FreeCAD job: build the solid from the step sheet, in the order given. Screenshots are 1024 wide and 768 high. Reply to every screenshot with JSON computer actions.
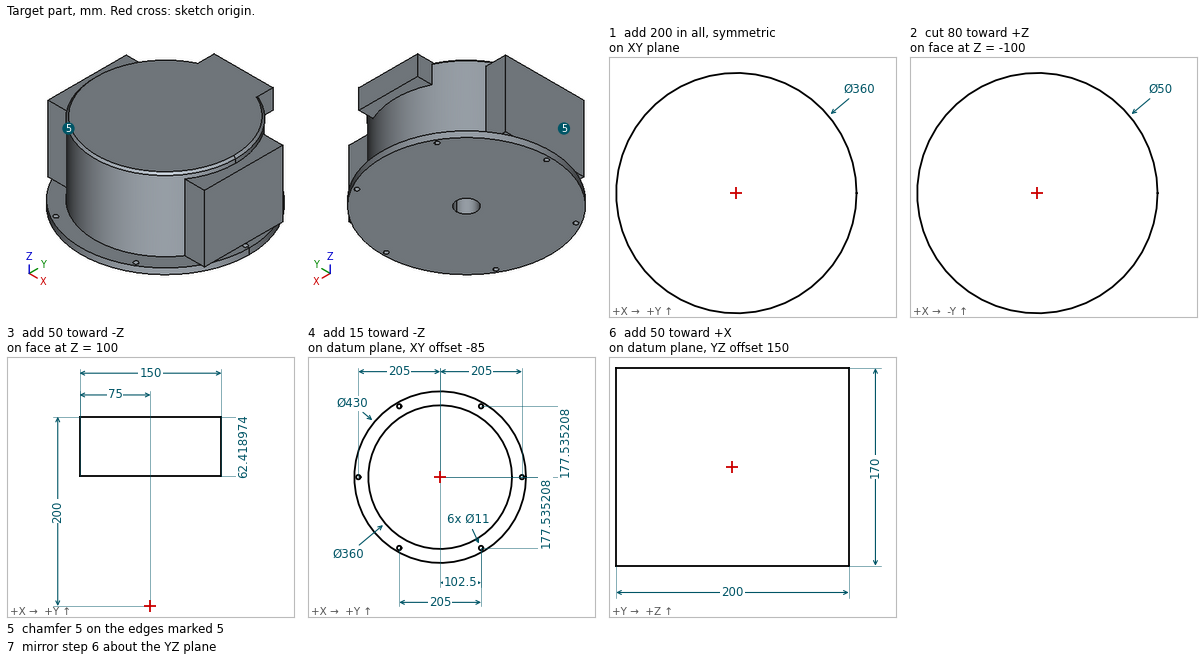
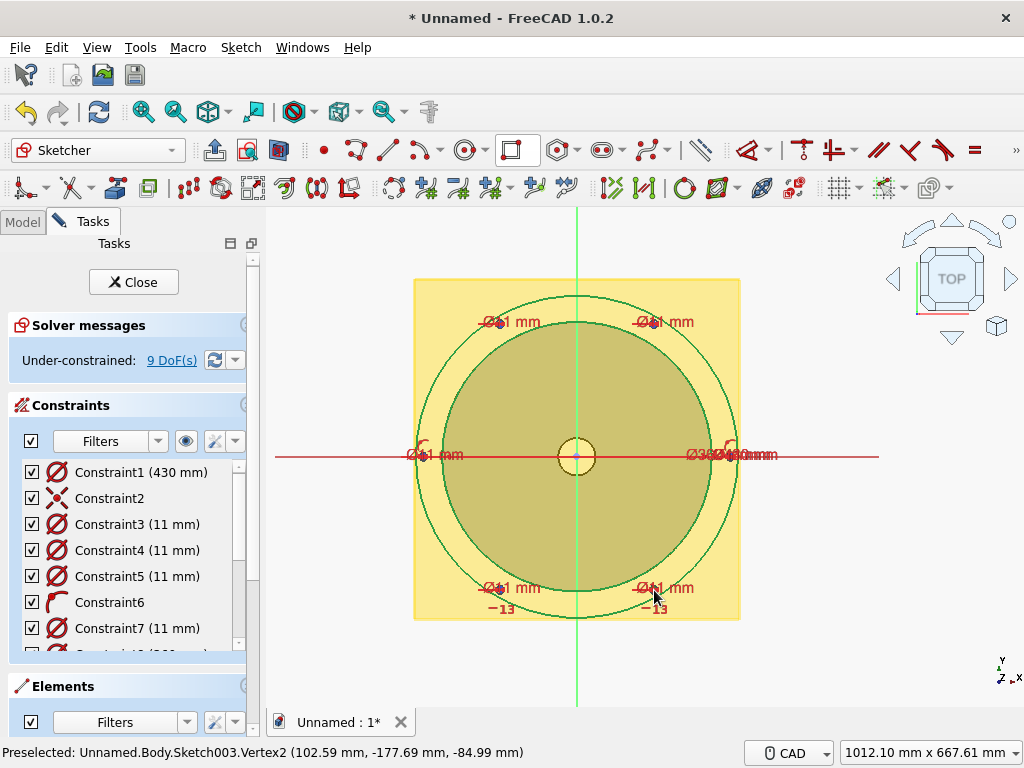
{"action": "left_click", "coordinate": [654, 324]}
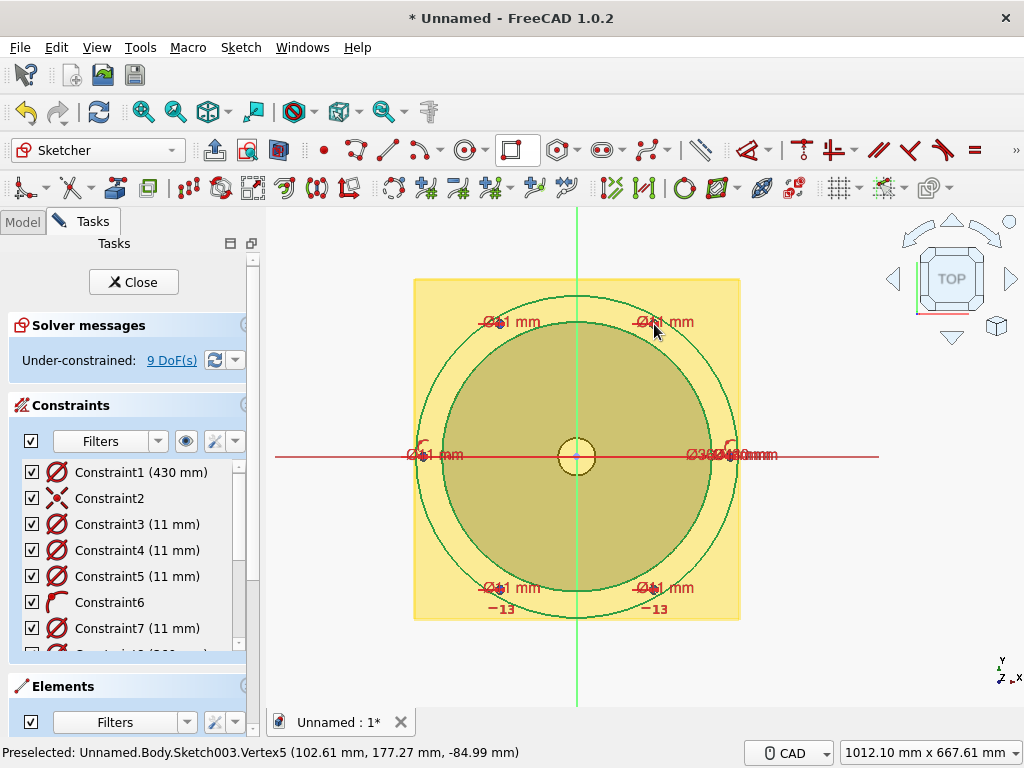
{"action": "key", "text": "v"}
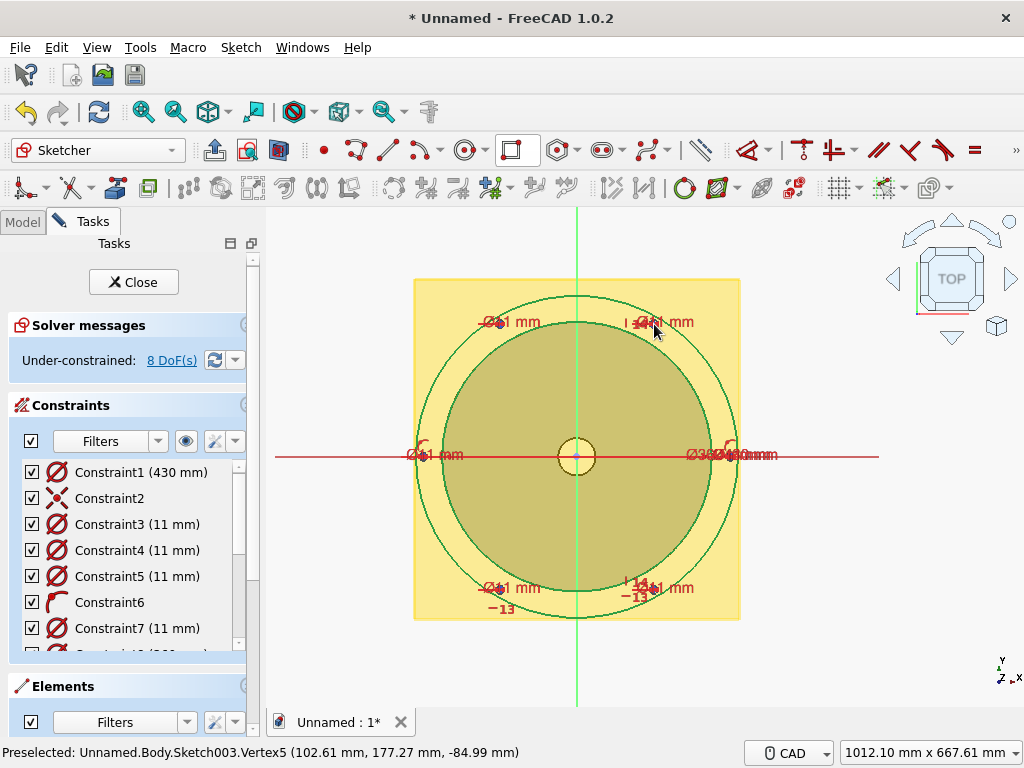
{"action": "left_click", "coordinate": [500, 590]}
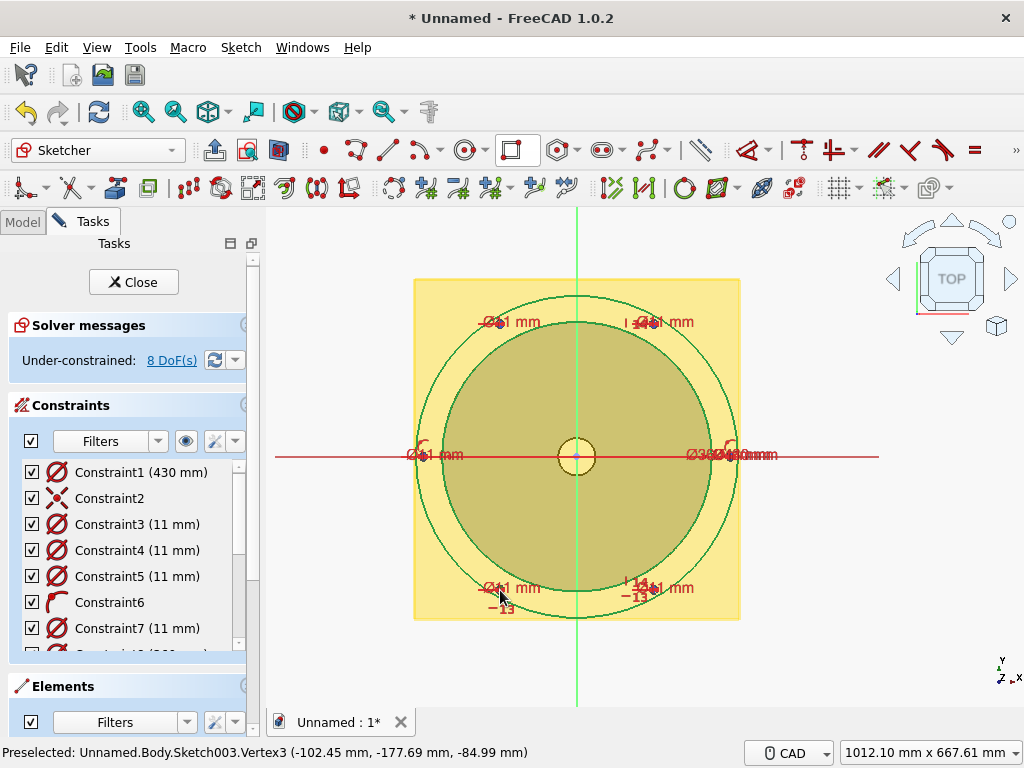
{"action": "left_click", "coordinate": [500, 324]}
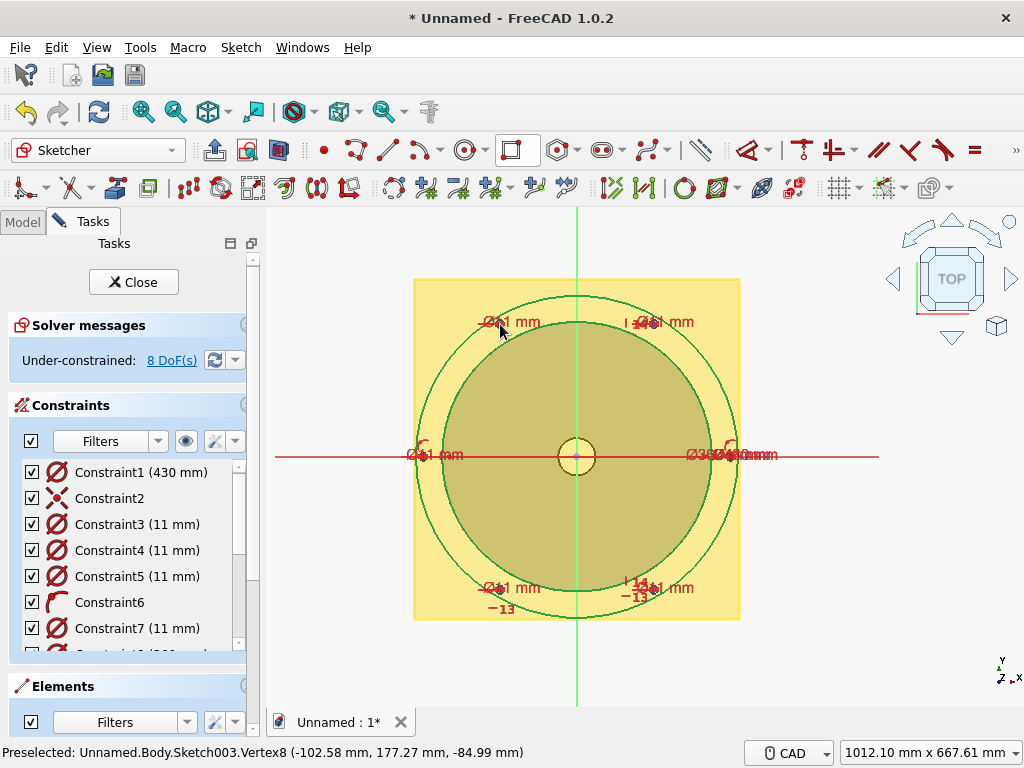
{"action": "left_click", "coordinate": [856, 150]}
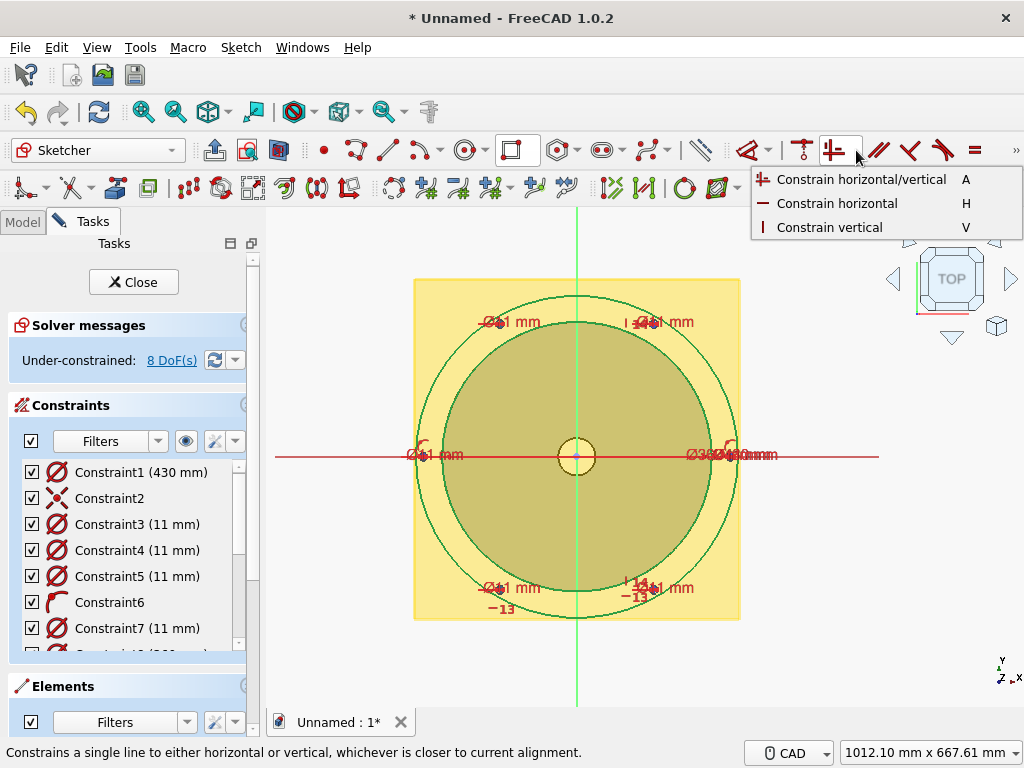
{"action": "left_click", "coordinate": [887, 227]}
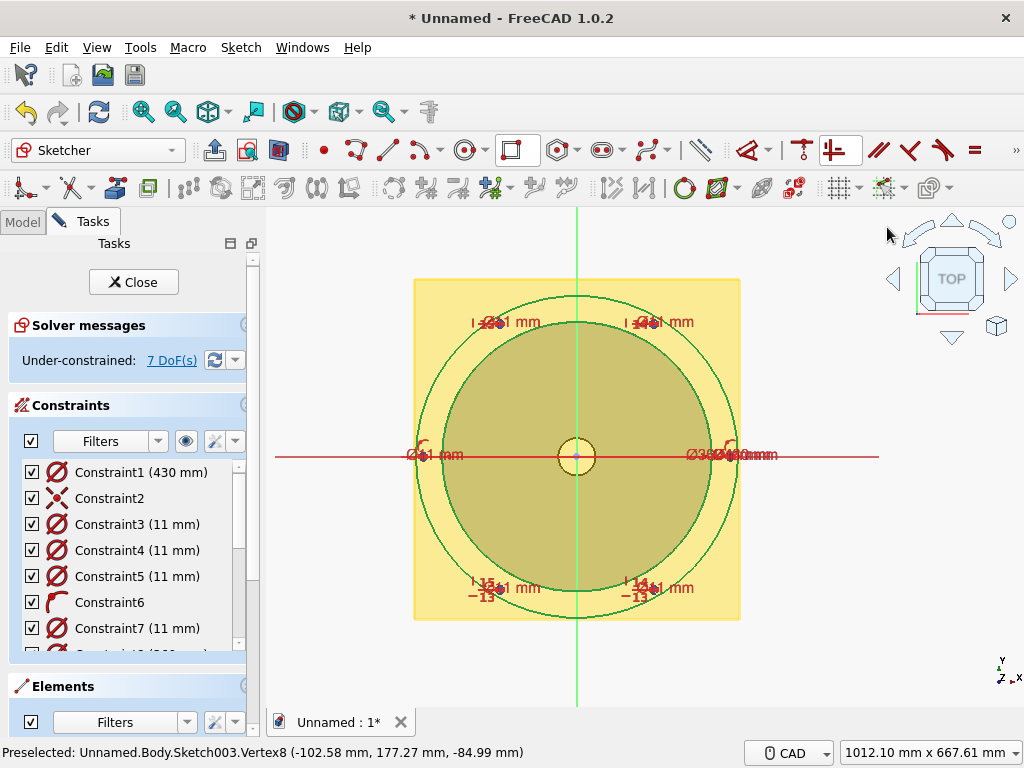
{"action": "left_click", "coordinate": [654, 324]}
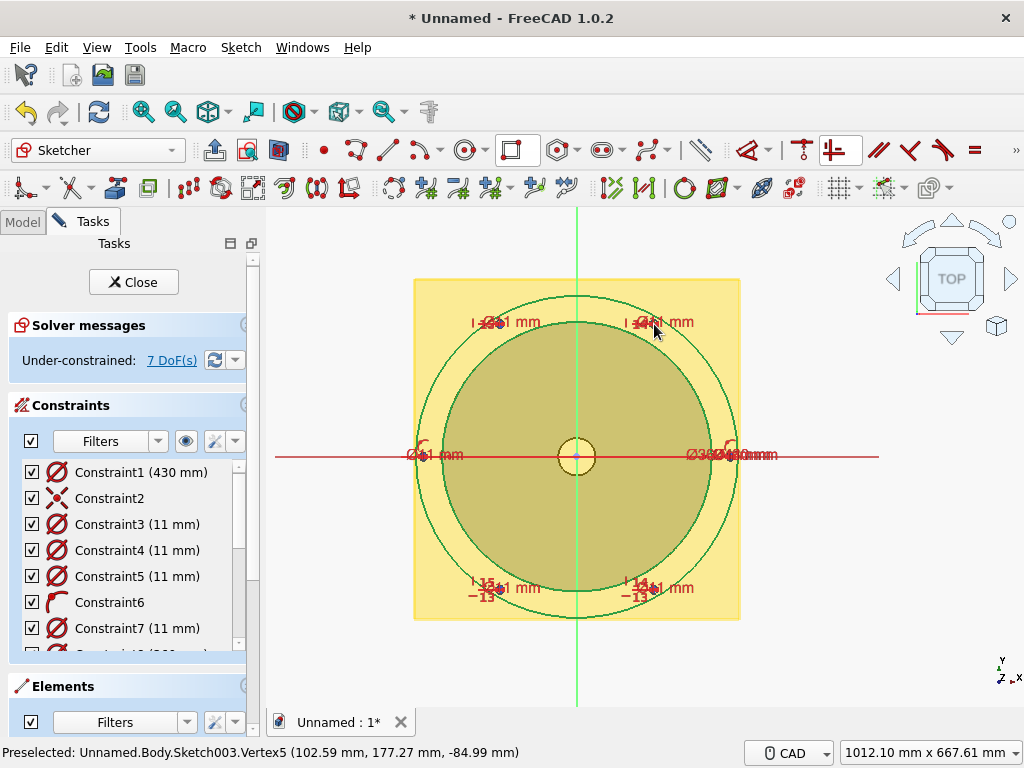
{"action": "left_click", "coordinate": [500, 324]}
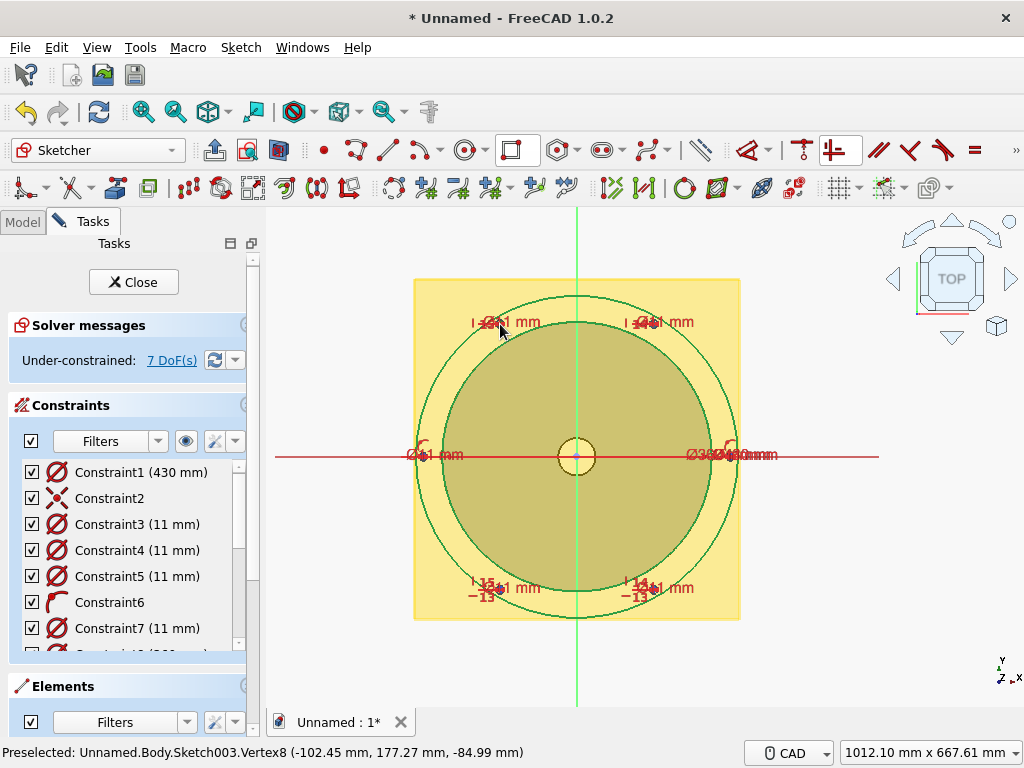
{"action": "key", "text": "h"}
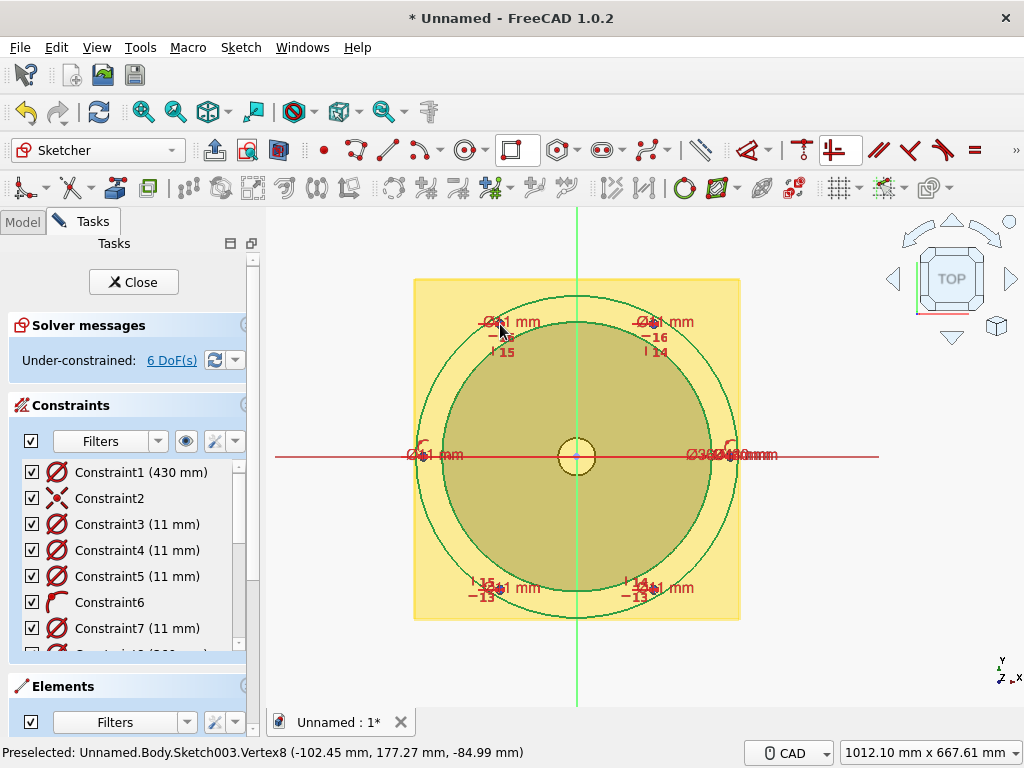
{"action": "left_click", "coordinate": [748, 150]}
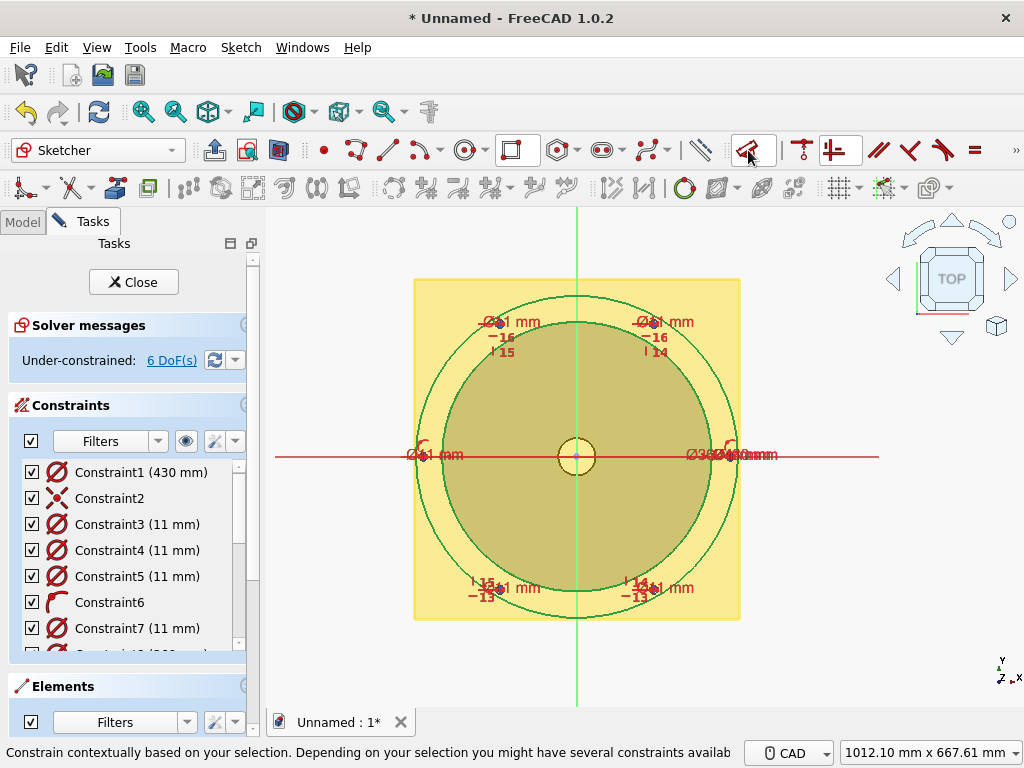
{"action": "left_click", "coordinate": [730, 457]}
{"action": "left_click", "coordinate": [654, 491]}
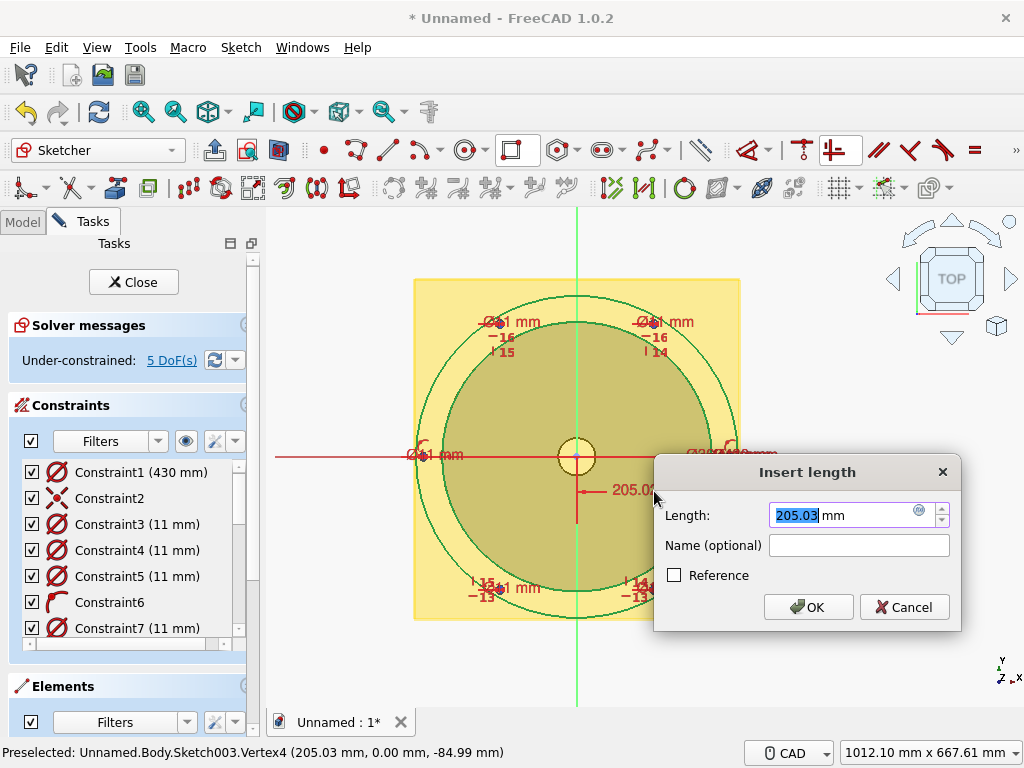
{"action": "type", "text": "205"}
{"action": "key", "text": "Return"}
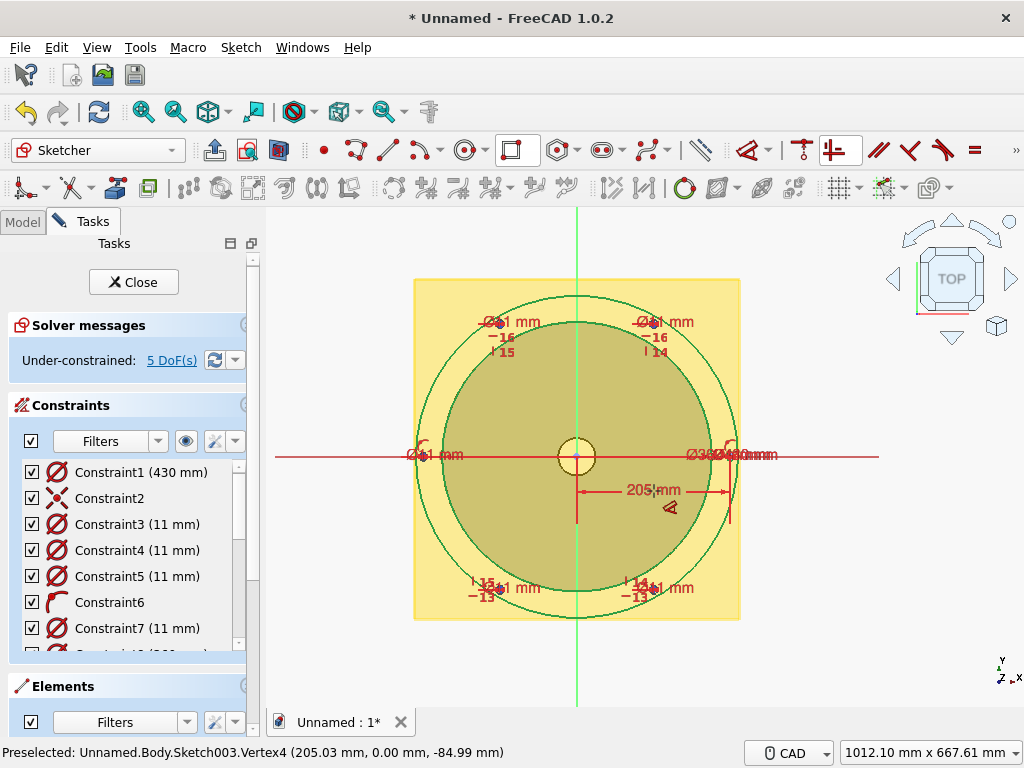
{"action": "left_click", "coordinate": [423, 457]}
{"action": "left_click", "coordinate": [500, 491]}